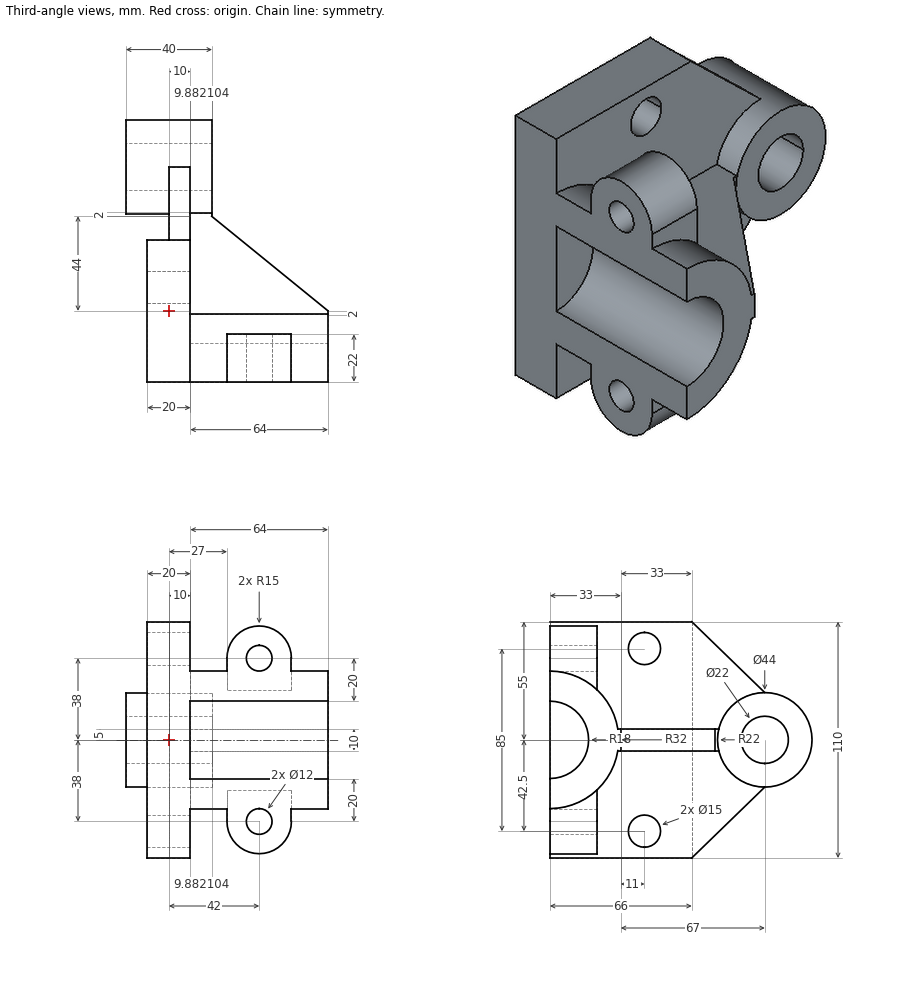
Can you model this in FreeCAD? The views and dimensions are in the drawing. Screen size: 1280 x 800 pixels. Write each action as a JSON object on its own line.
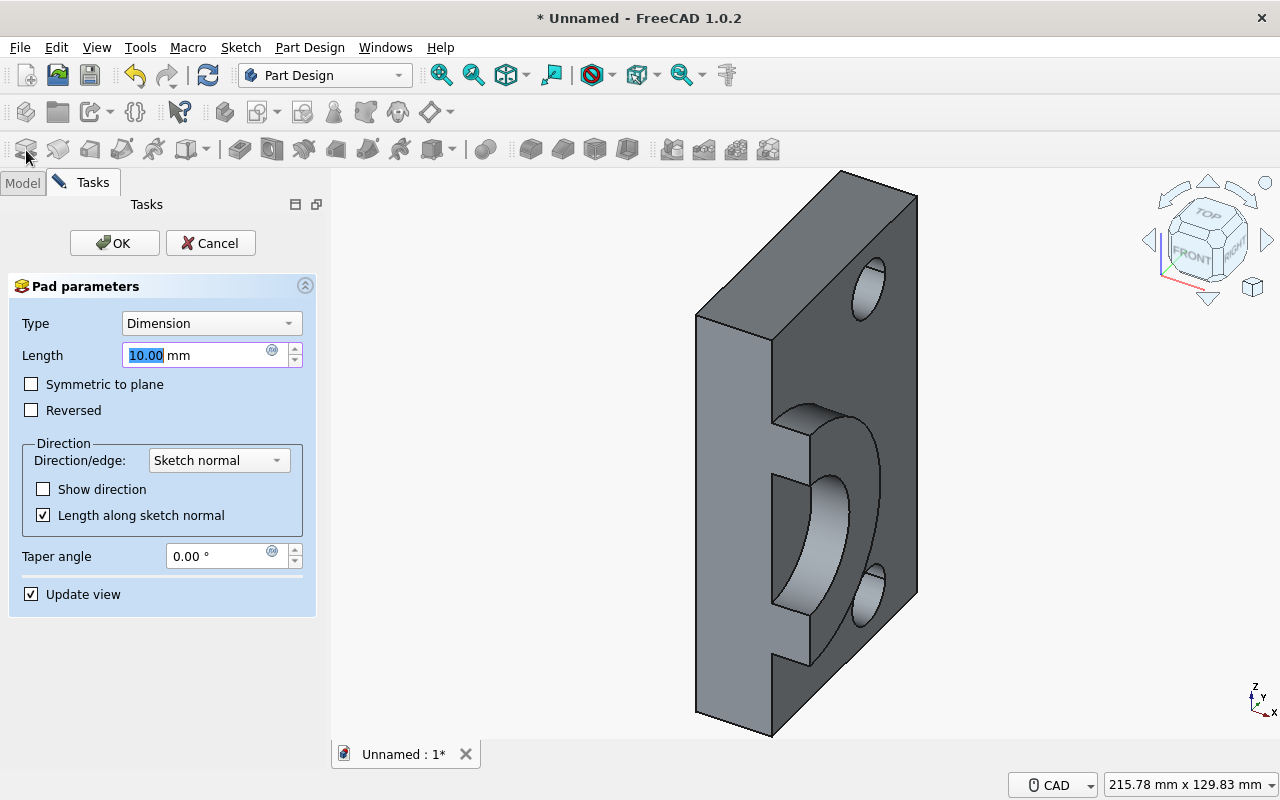
{"action": "type", "text": "64"}
{"action": "key", "text": "Tab"}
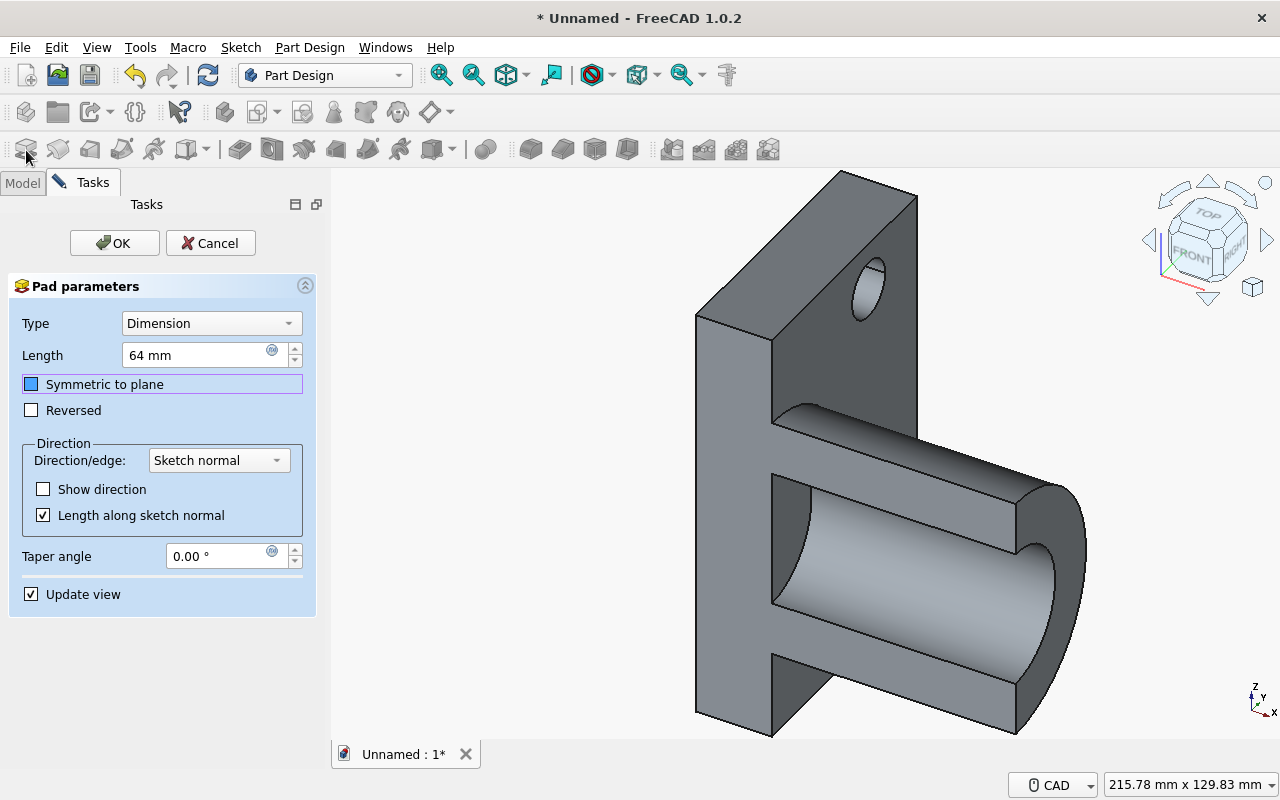
{"action": "left_click", "coordinate": [115, 243]}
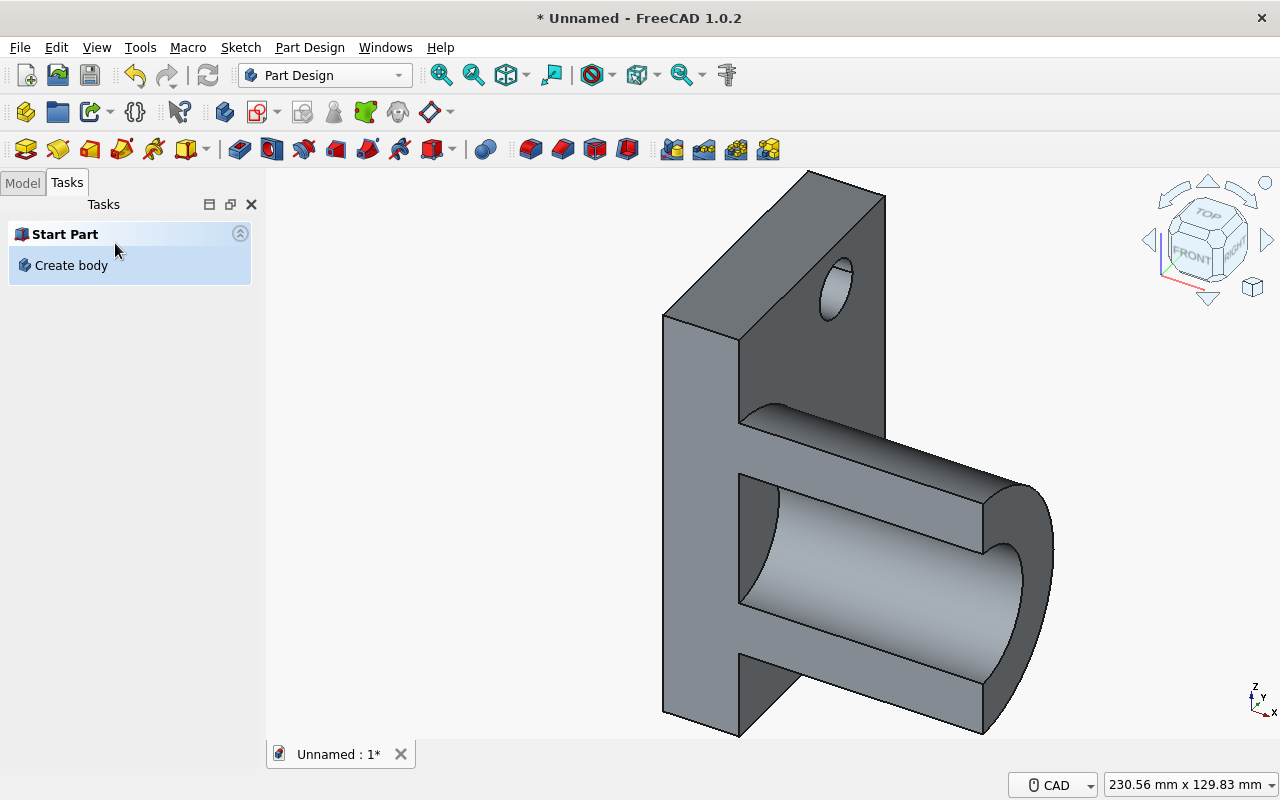
{"action": "left_click", "coordinate": [442, 76]}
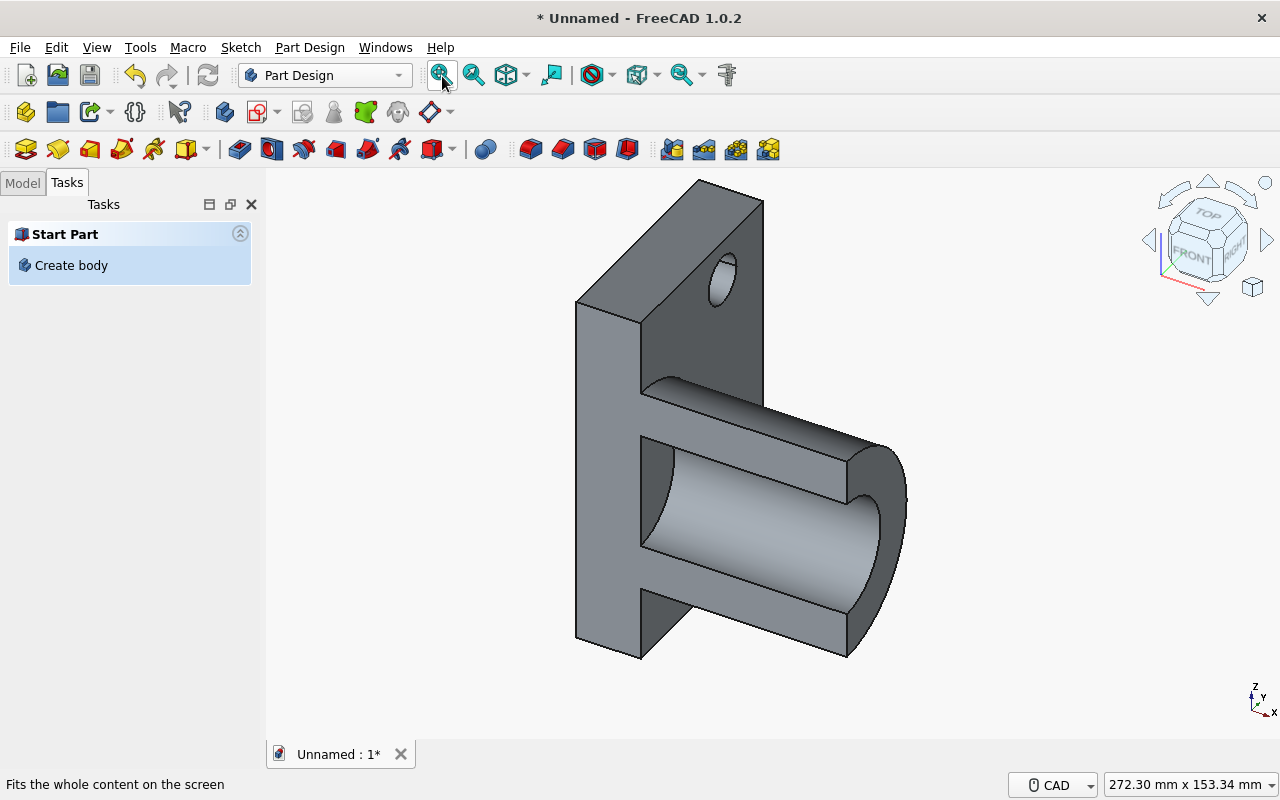
{"action": "left_click", "coordinate": [595, 331]}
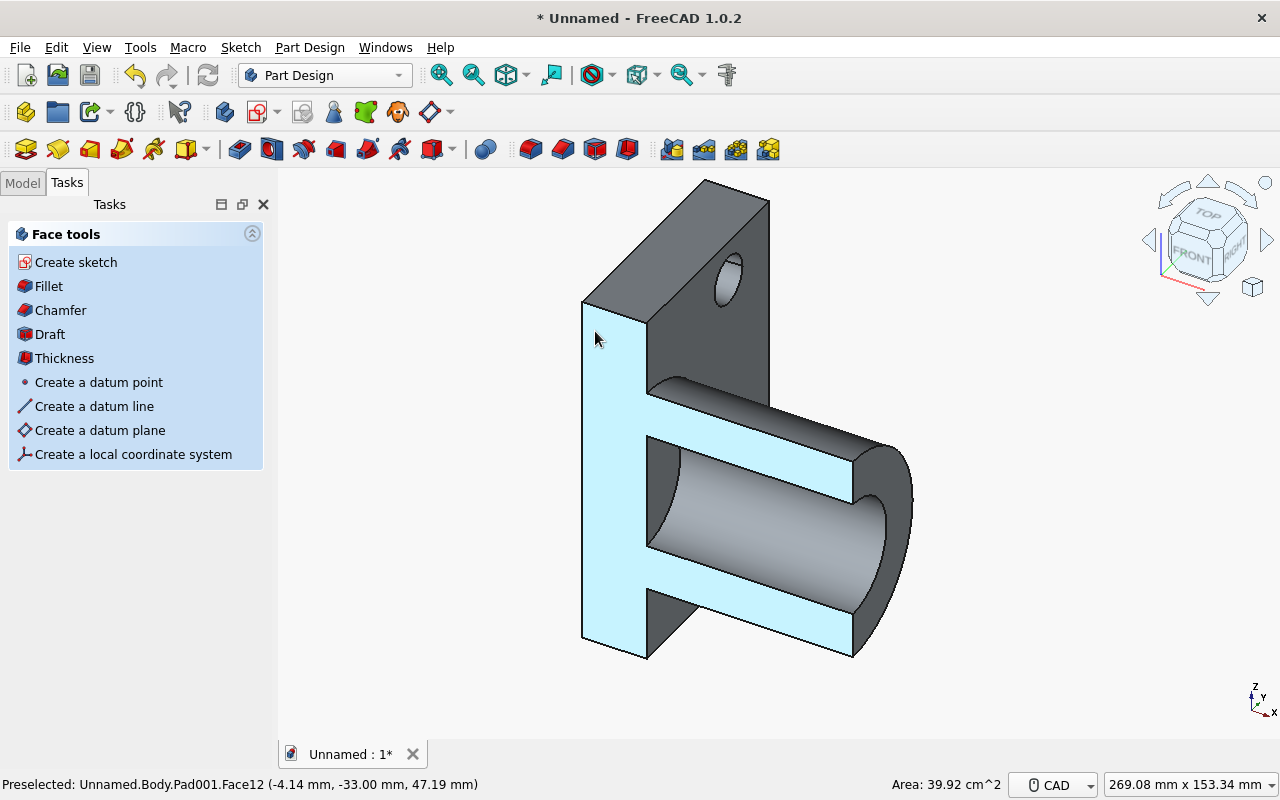
{"action": "left_click", "coordinate": [258, 112]}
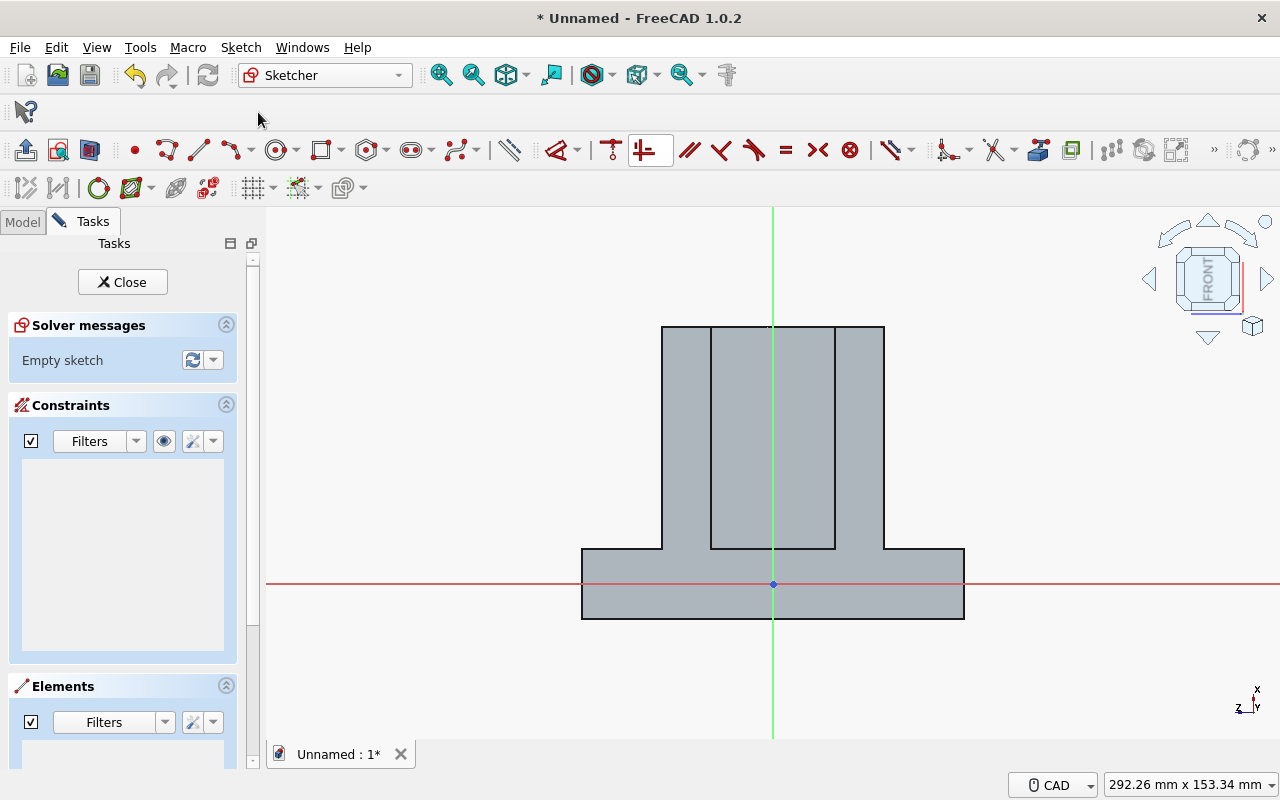
{"action": "scroll", "coordinate": [912, 510], "scroll_direction": "up", "scroll_amount": 2}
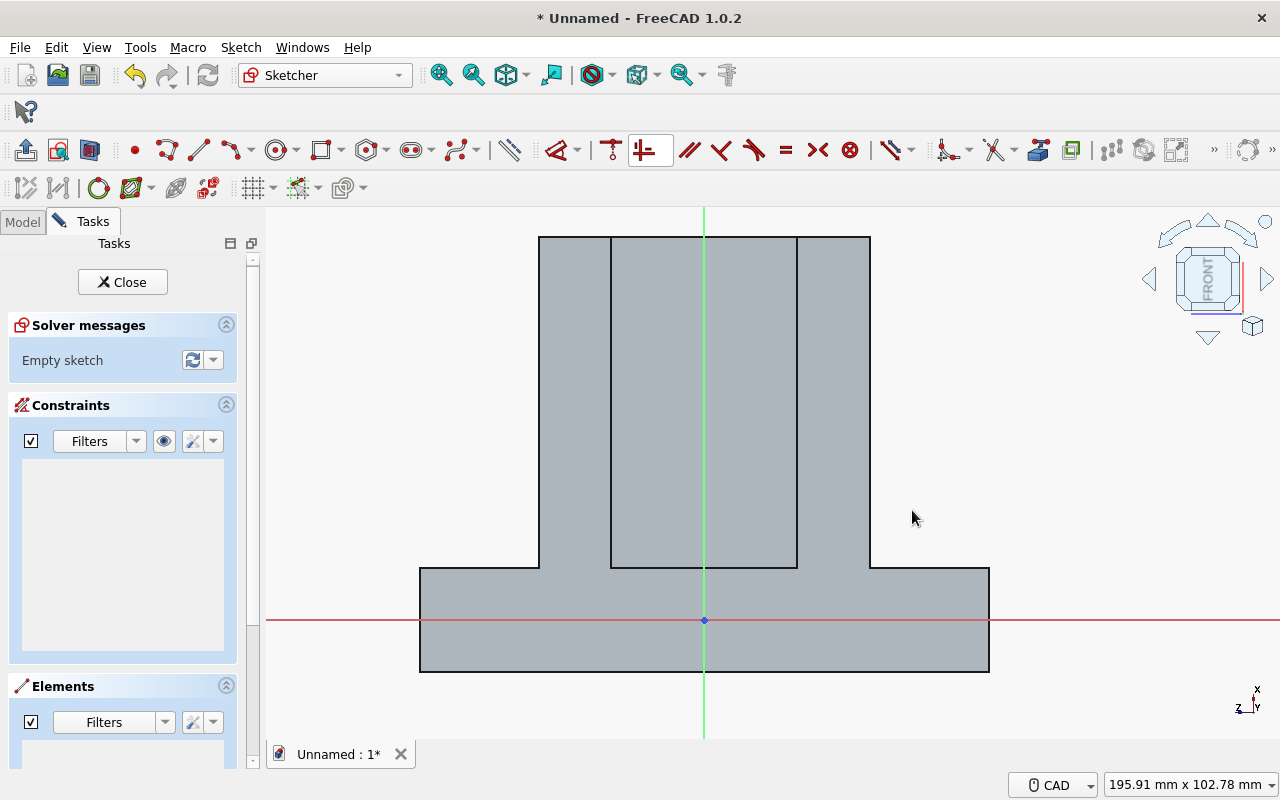
{"action": "left_click", "coordinate": [168, 150]}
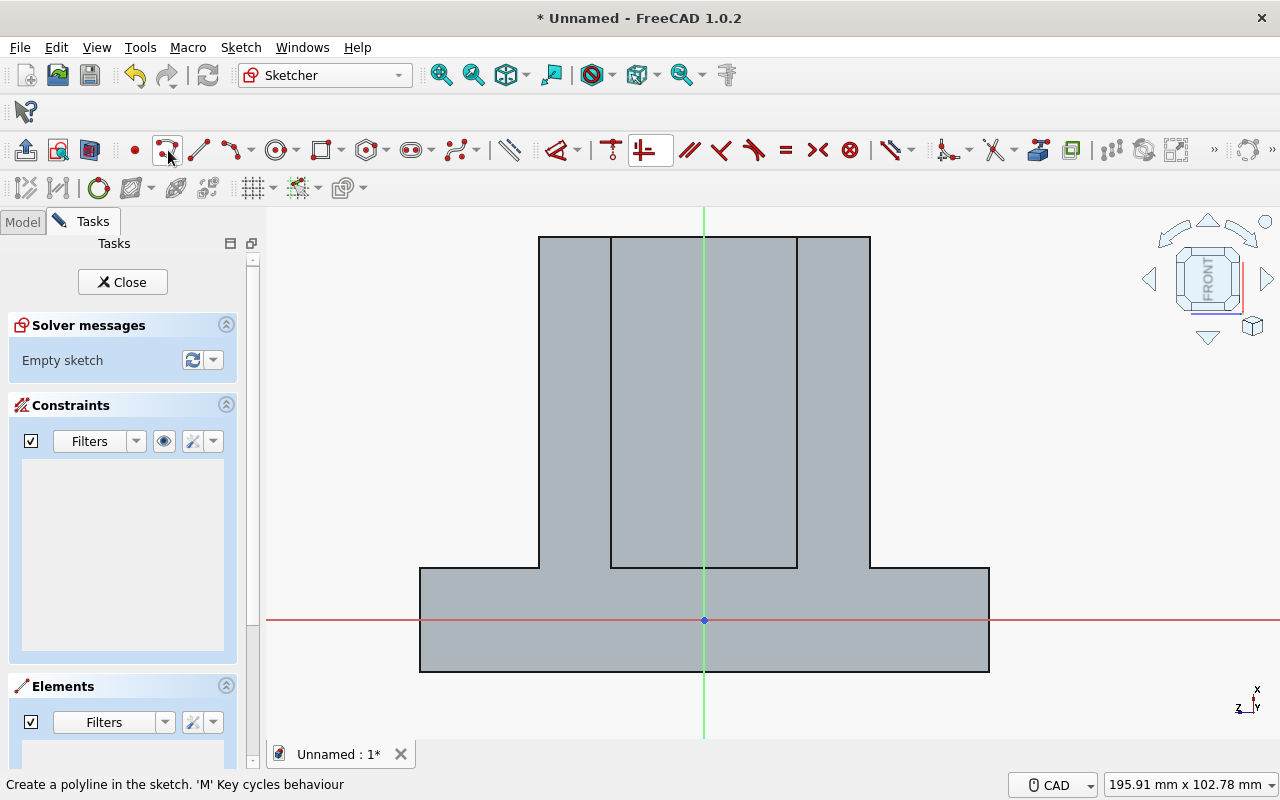
{"action": "left_click", "coordinate": [508, 480]}
{"action": "left_click", "coordinate": [611, 480]}
{"action": "left_click", "coordinate": [611, 325]}
{"action": "left_click", "coordinate": [508, 325]}
{"action": "right_click", "coordinate": [508, 325]}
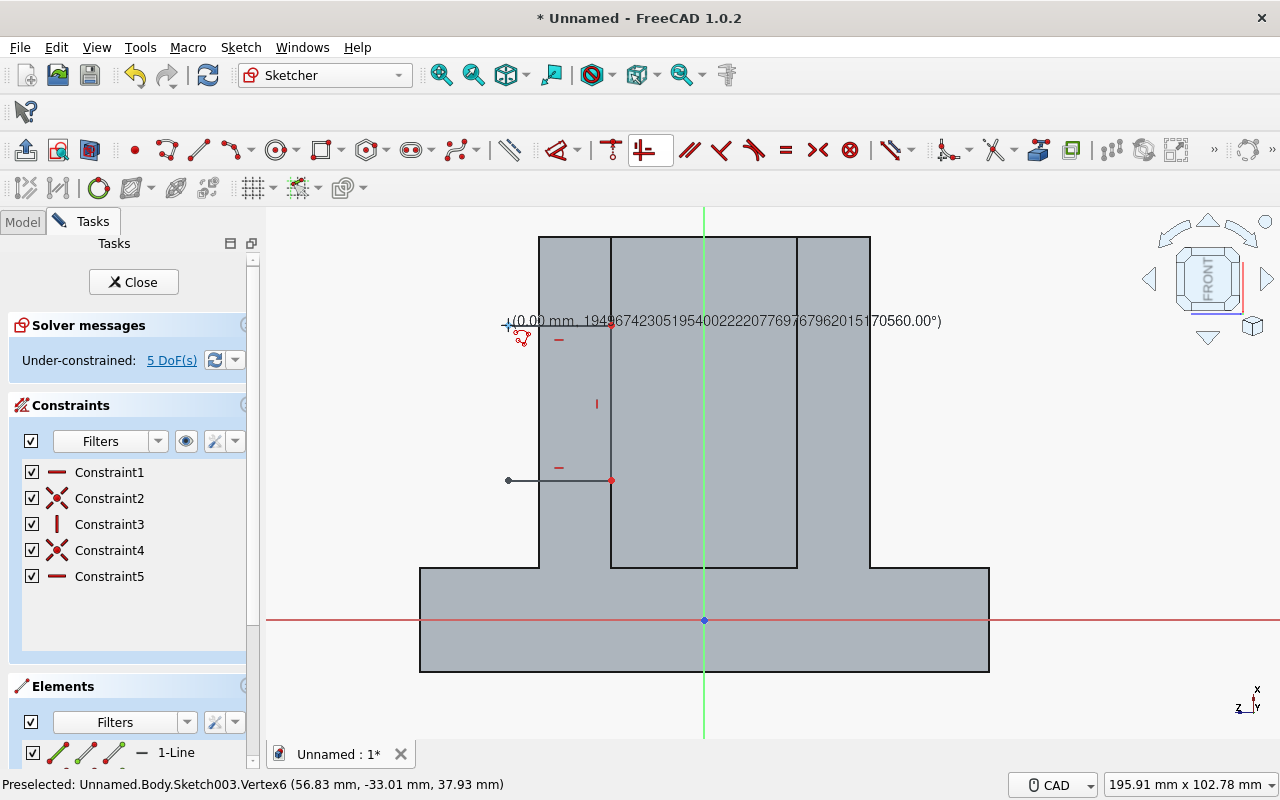
{"action": "key", "text": "g 3 a"}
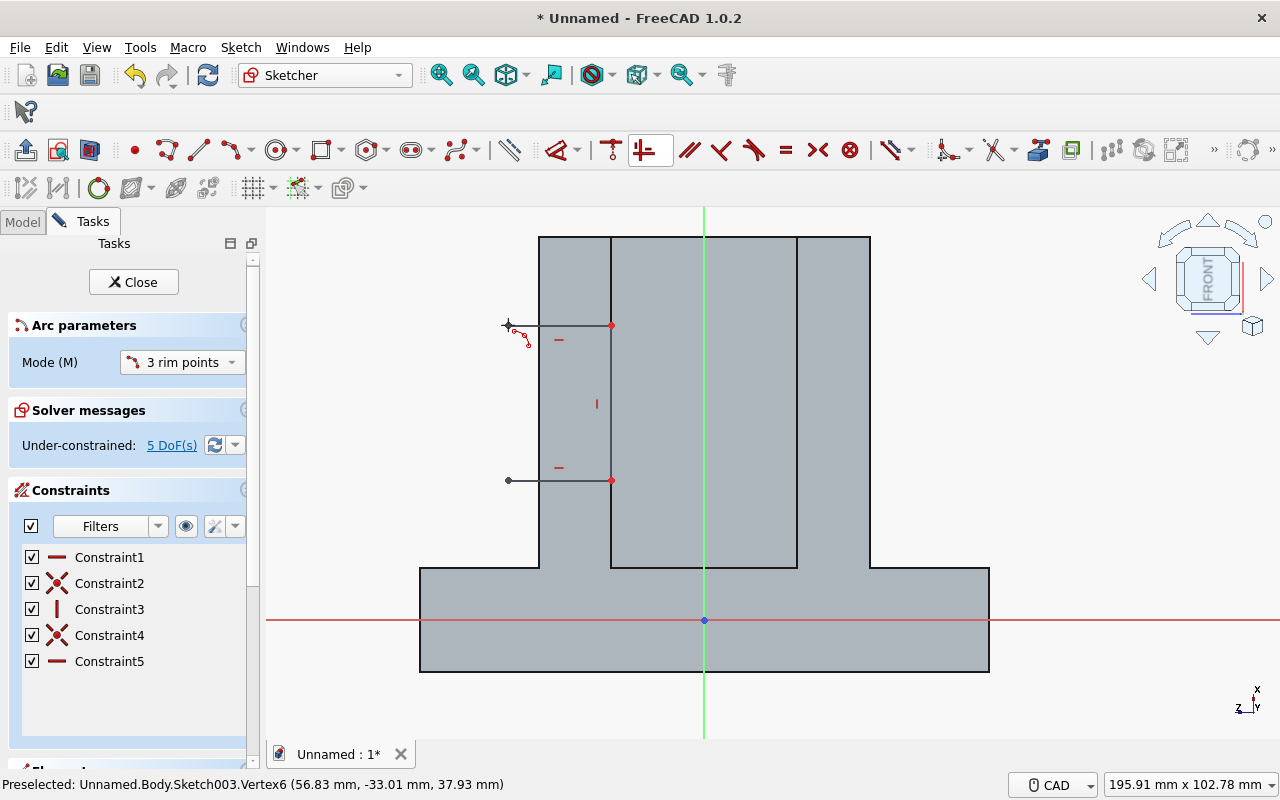
{"action": "left_click", "coordinate": [508, 326]}
{"action": "left_click", "coordinate": [508, 481]}
{"action": "left_click", "coordinate": [430, 403]}